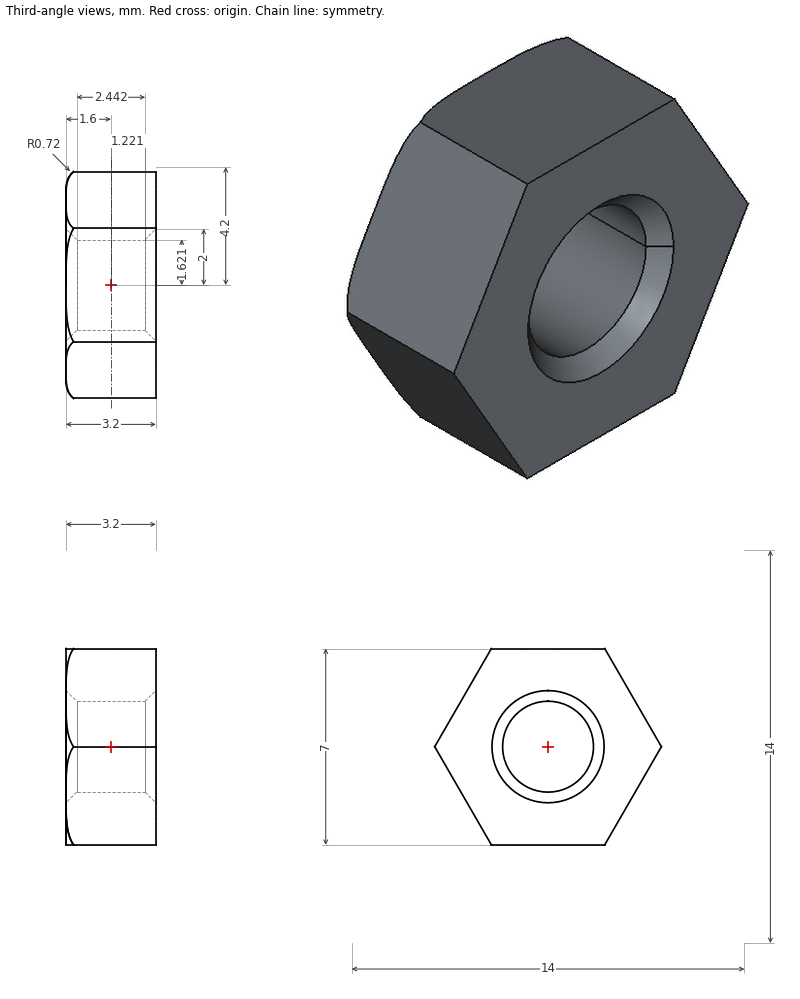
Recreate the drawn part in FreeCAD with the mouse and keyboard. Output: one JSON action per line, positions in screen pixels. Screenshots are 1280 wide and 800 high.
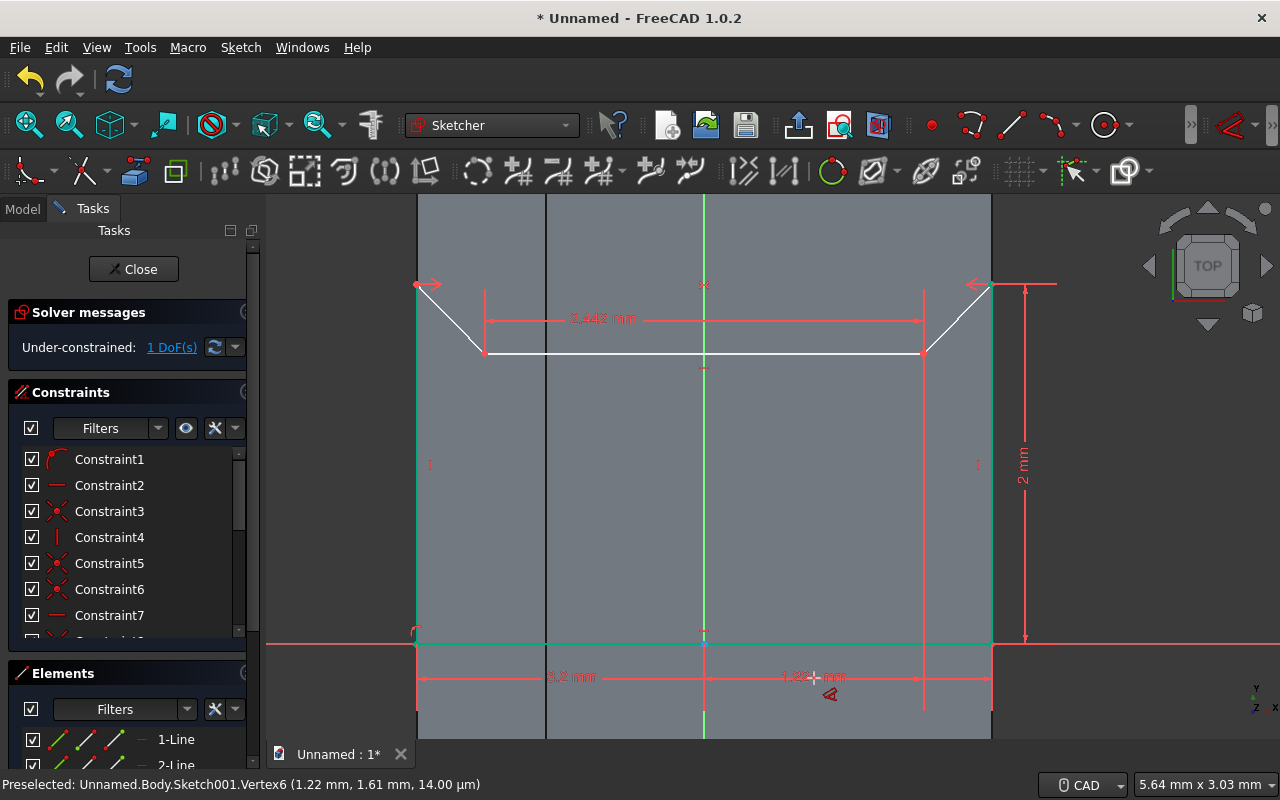
{"action": "left_click", "coordinate": [924, 354]}
{"action": "left_click", "coordinate": [958, 499]}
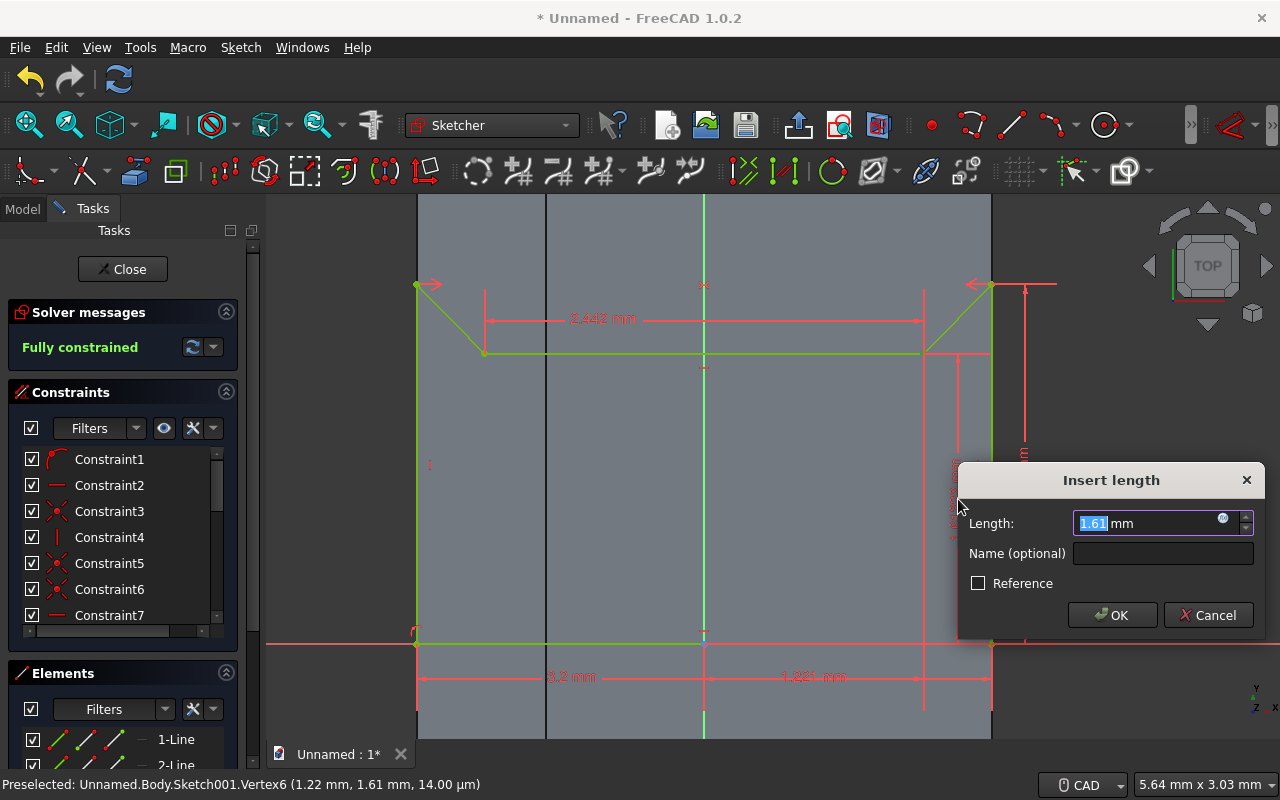
{"action": "type", "text": "1.621"}
{"action": "key", "text": "Return"}
{"action": "key", "text": "Escape"}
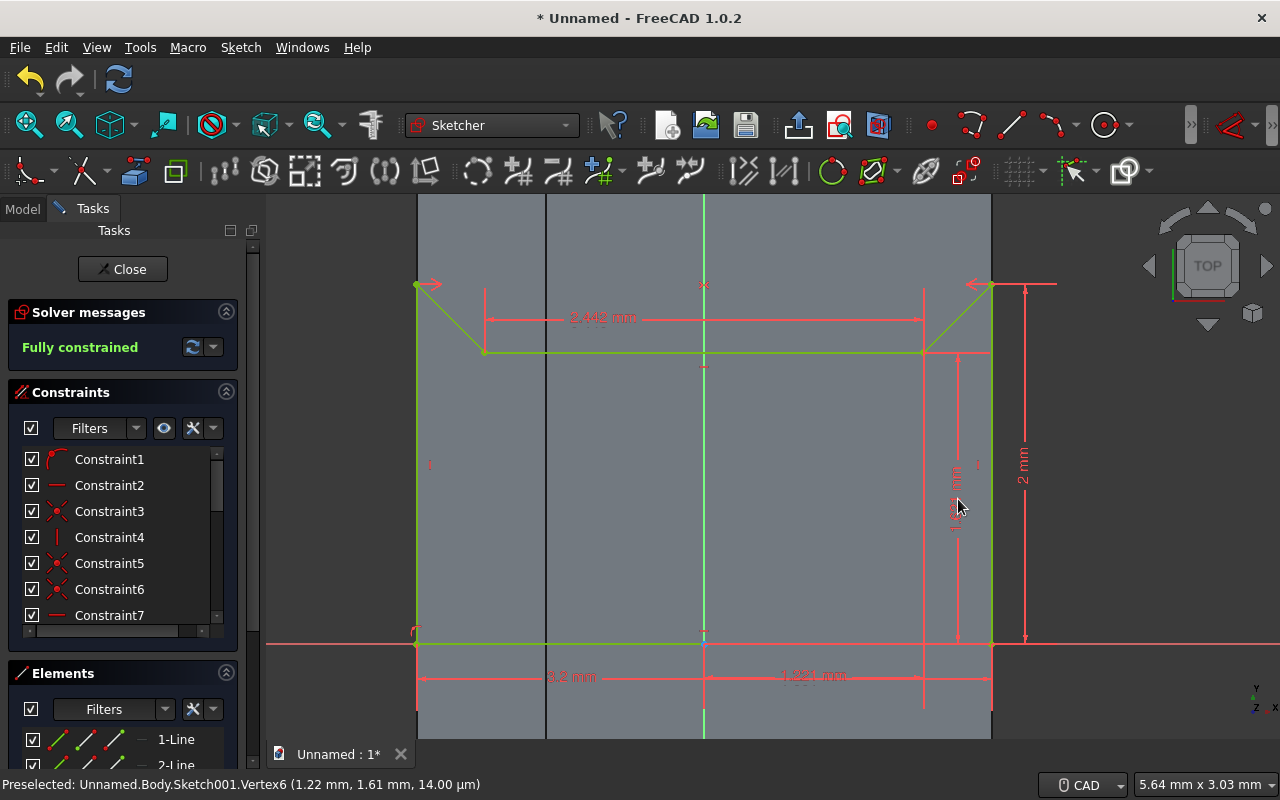
{"action": "left_click", "coordinate": [123, 269]}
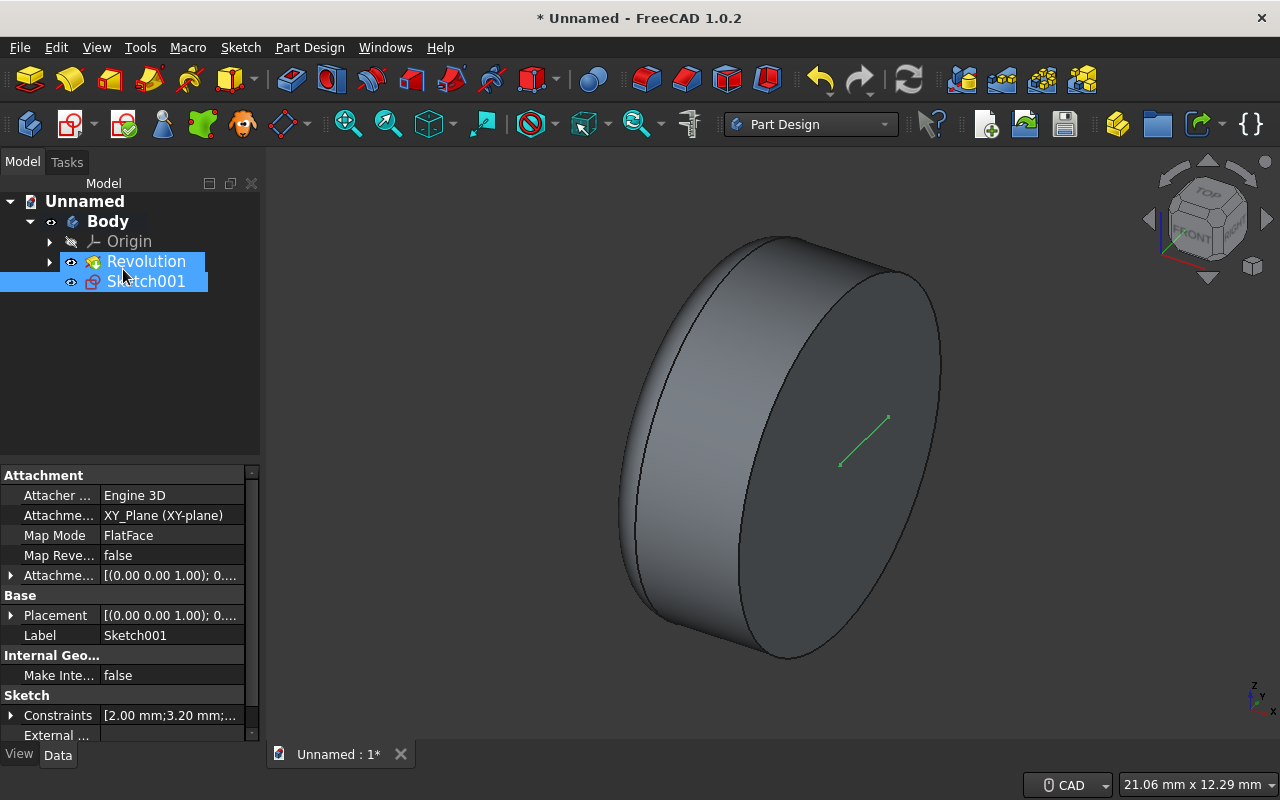
{"action": "left_click", "coordinate": [372, 80]}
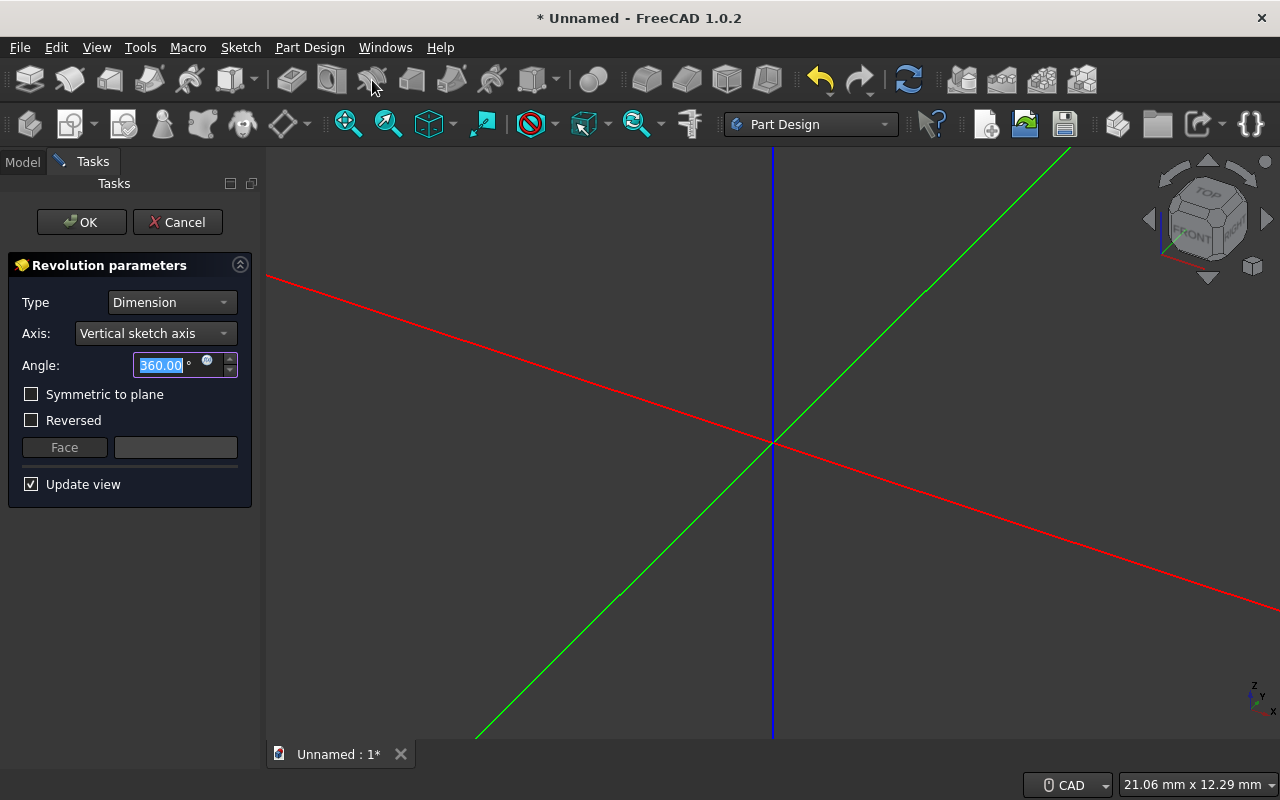
{"action": "left_click", "coordinate": [156, 334]}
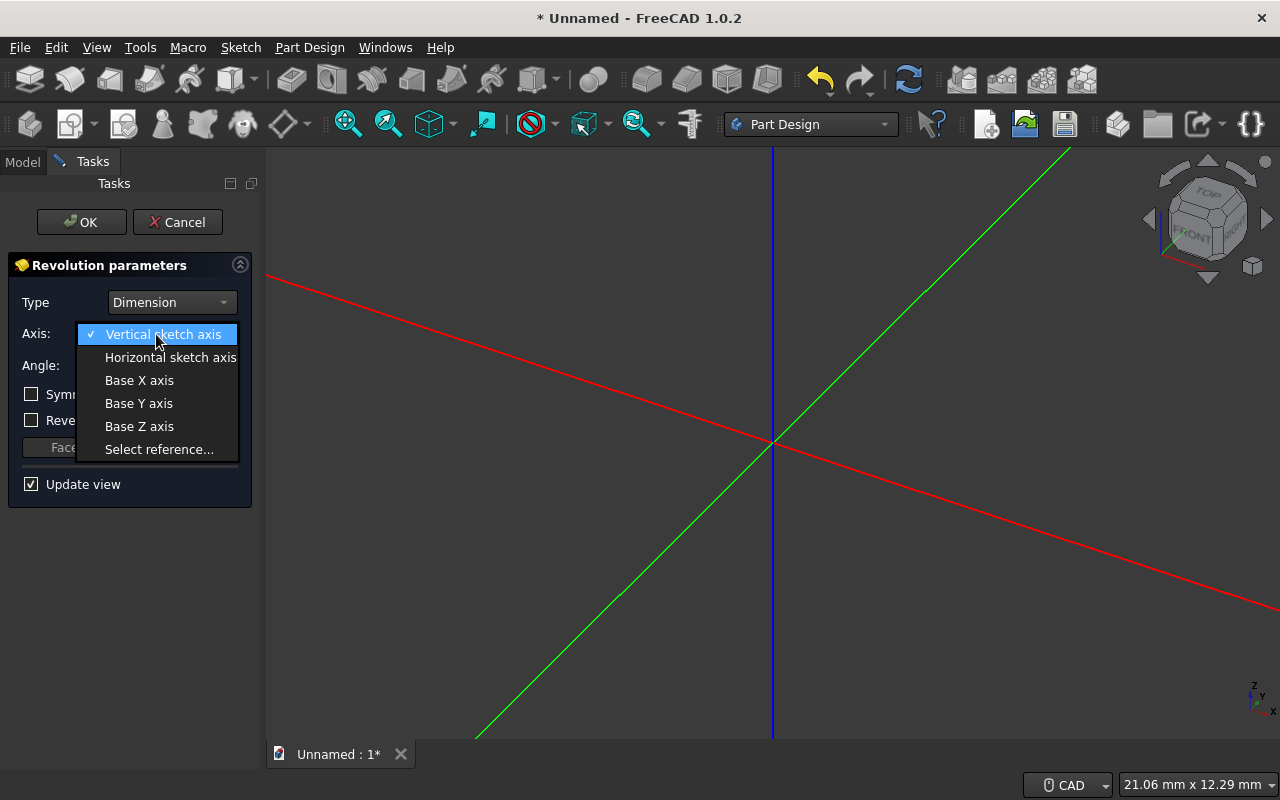
{"action": "left_click", "coordinate": [156, 358]}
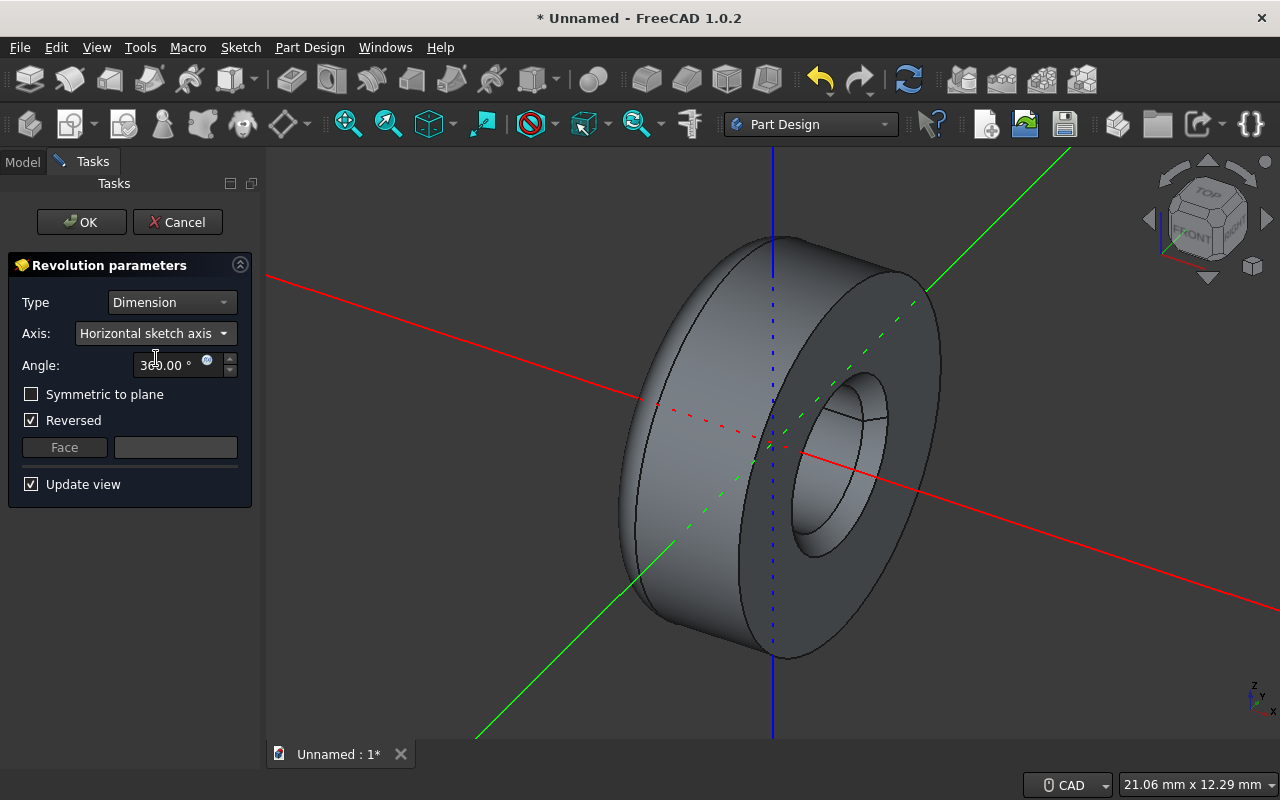
{"action": "left_click", "coordinate": [82, 222]}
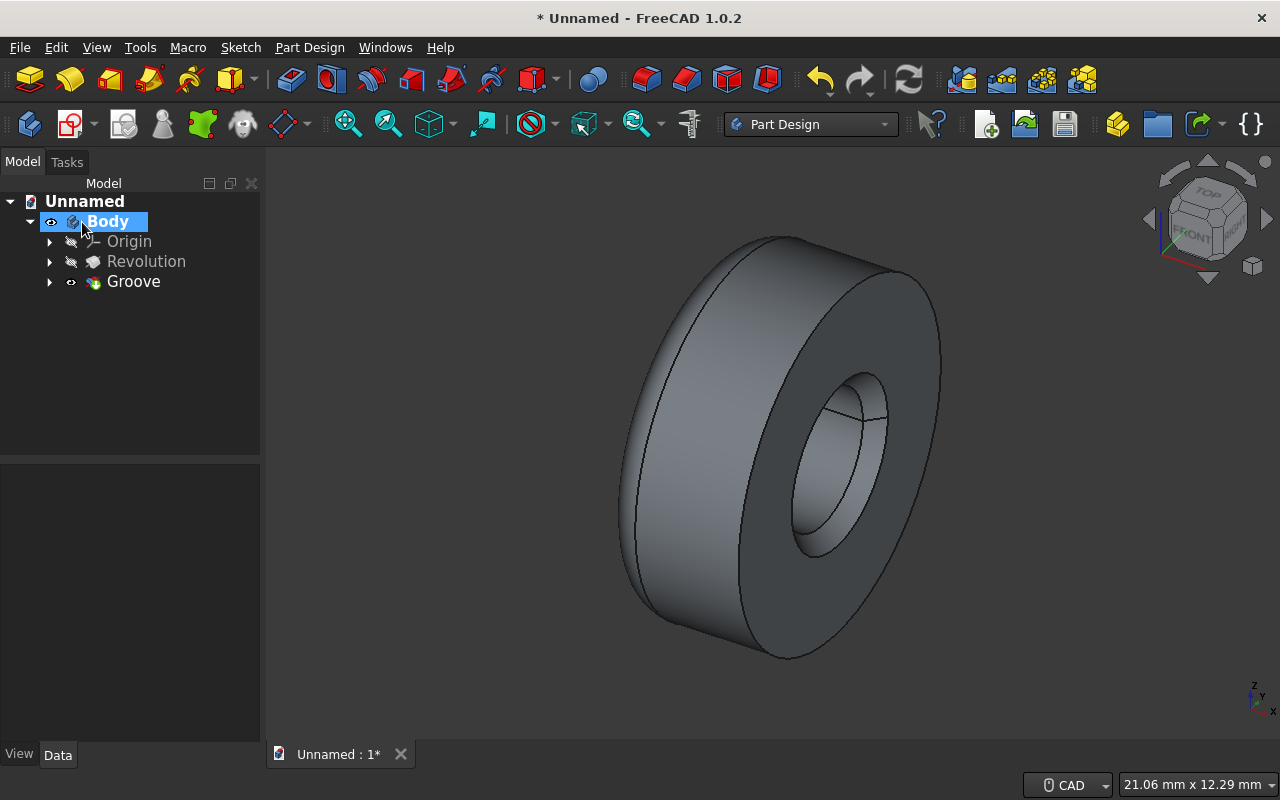
{"action": "left_click", "coordinate": [70, 124]}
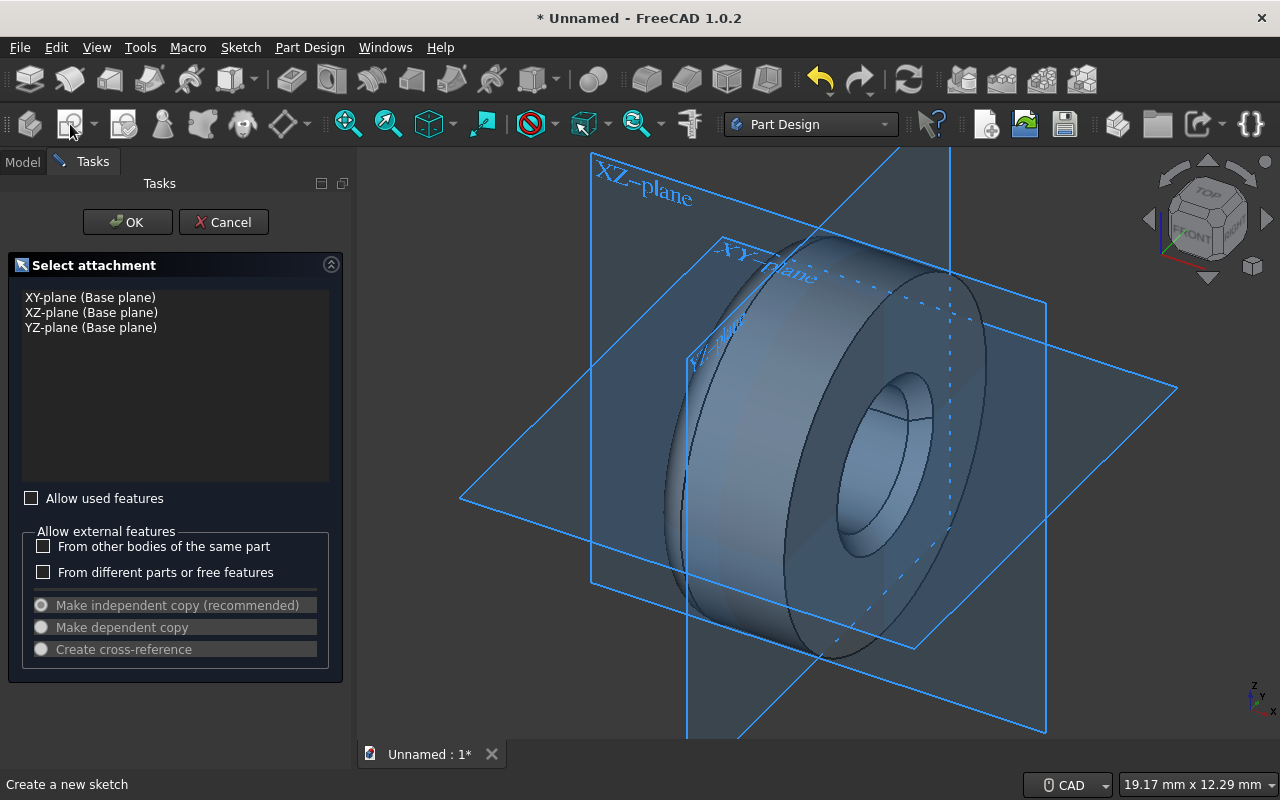
{"action": "left_click", "coordinate": [82, 328]}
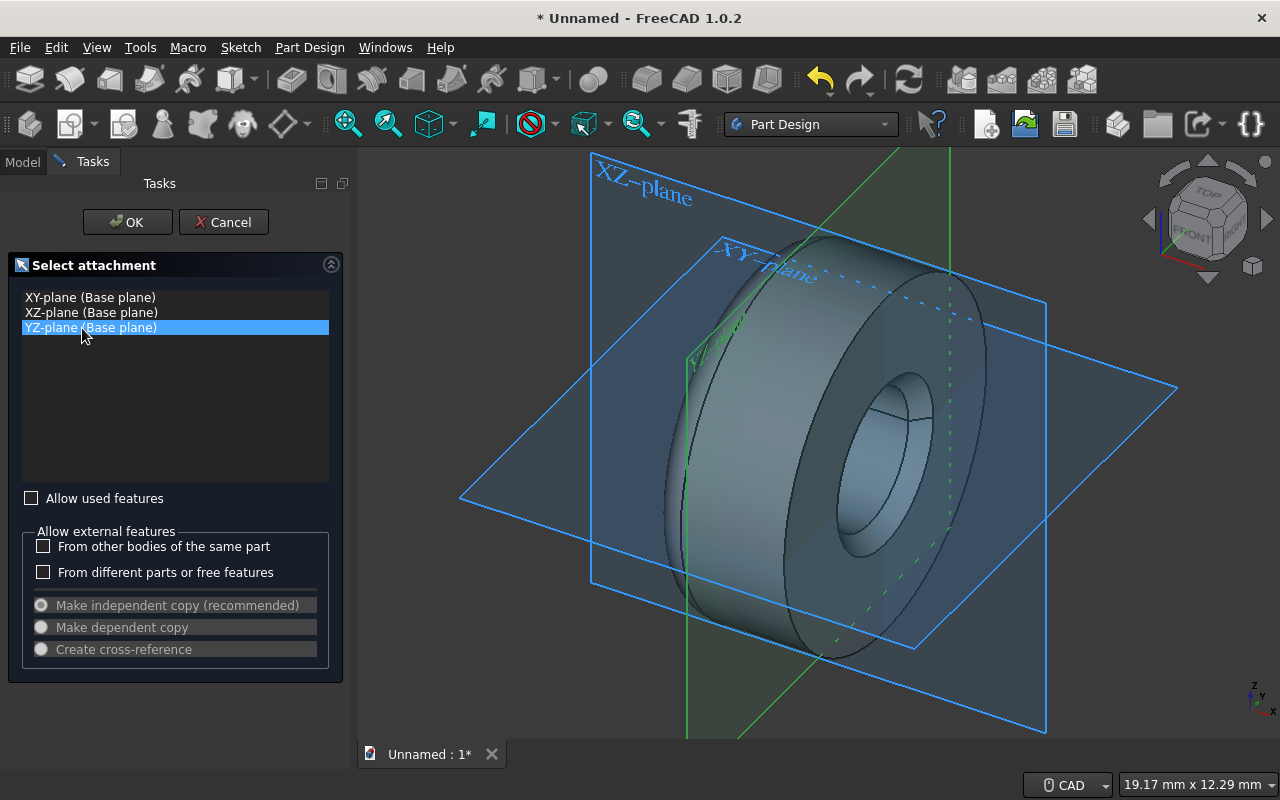
{"action": "left_click", "coordinate": [128, 222]}